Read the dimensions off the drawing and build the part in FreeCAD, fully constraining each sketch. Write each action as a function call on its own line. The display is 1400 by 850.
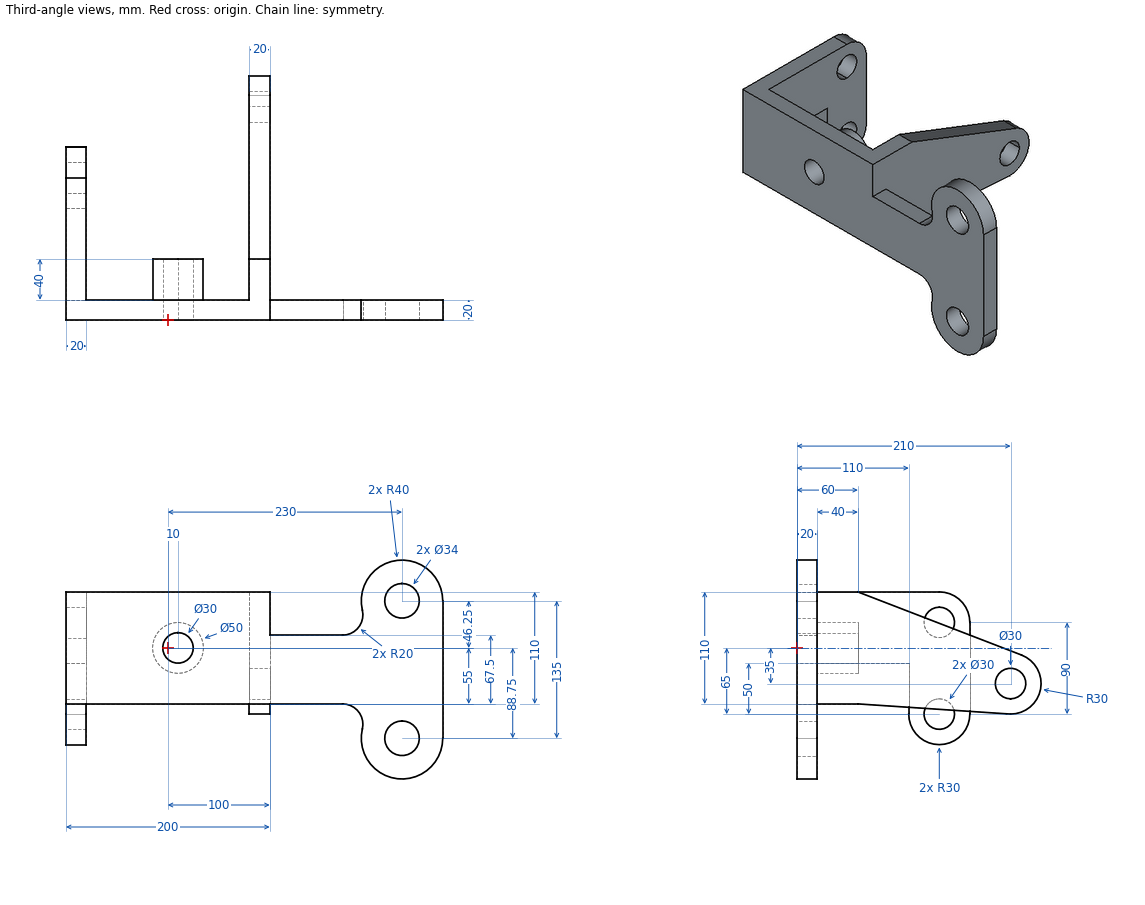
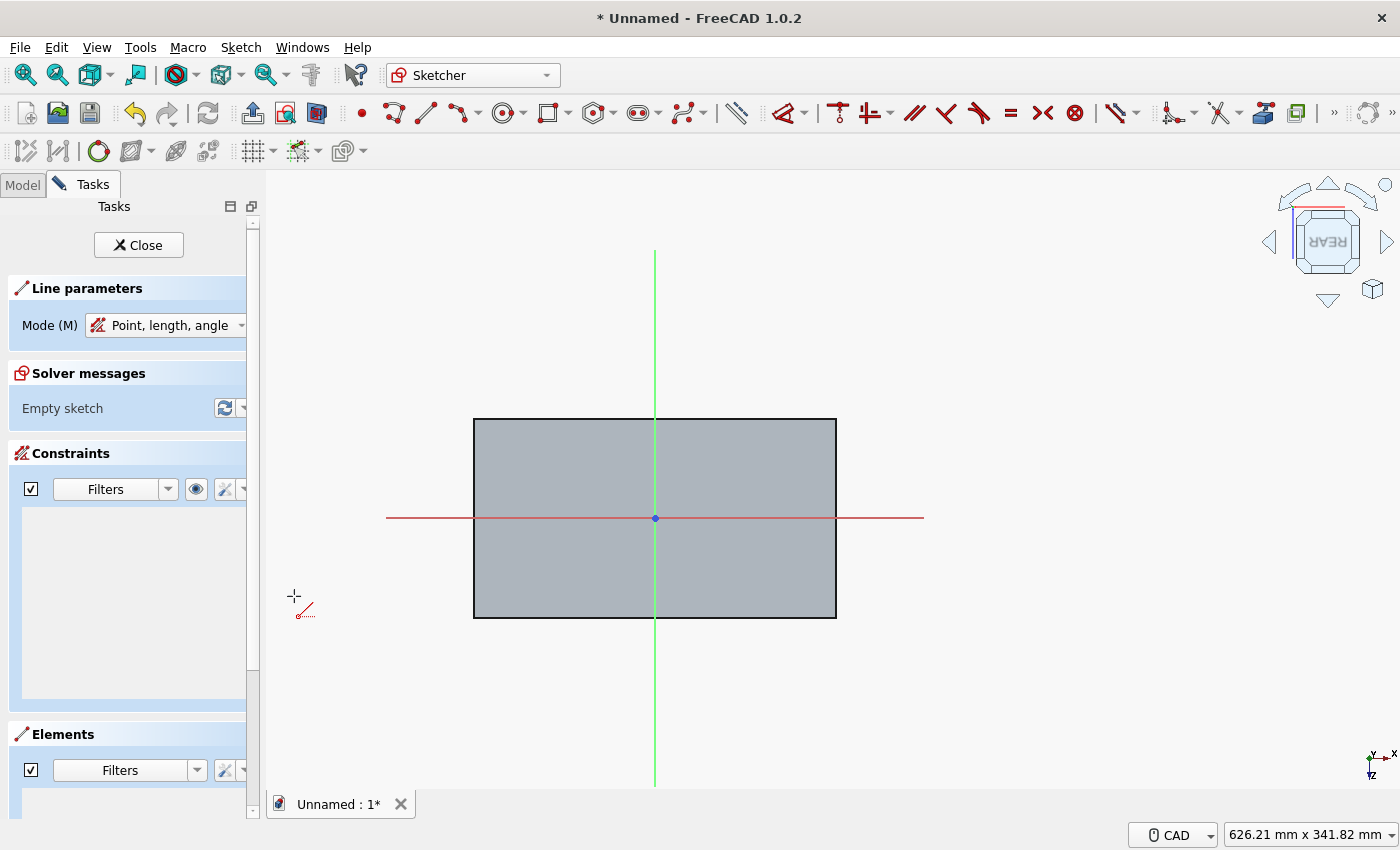
click(1144, 602)
click(1144, 357)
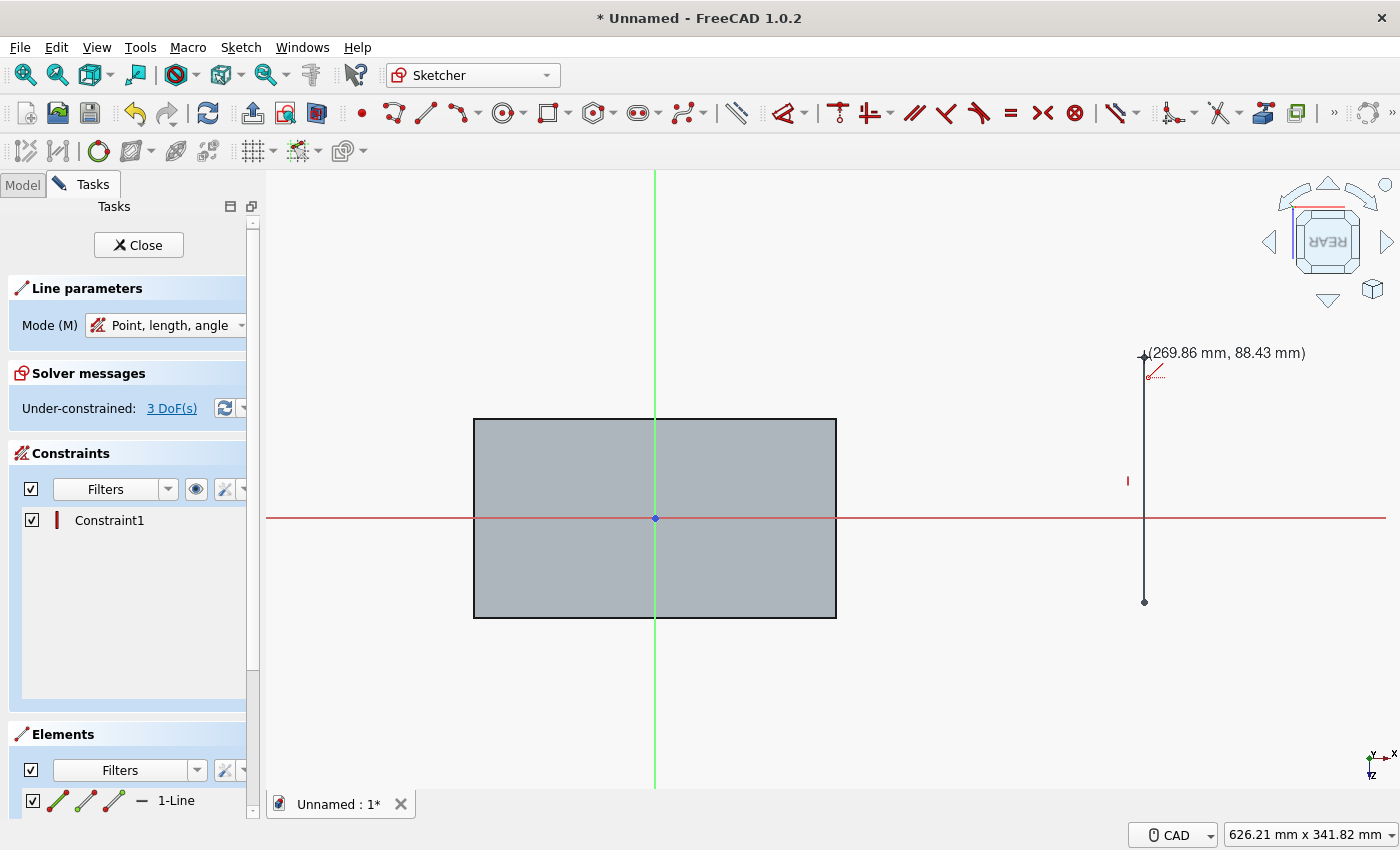
key(g)
key(m)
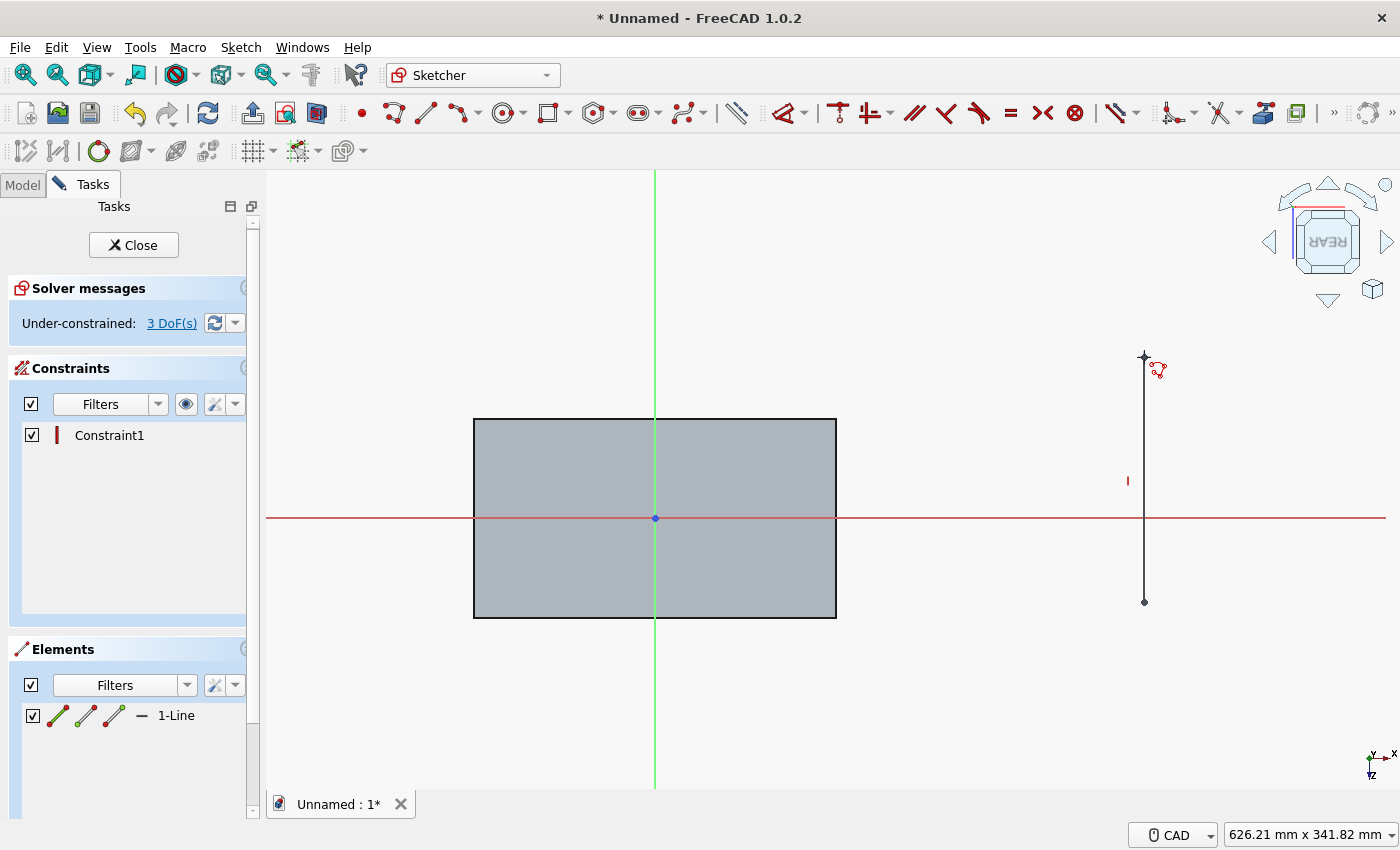
click(966, 419)
click(836, 419)
click(836, 541)
click(966, 541)
right_click(966, 541)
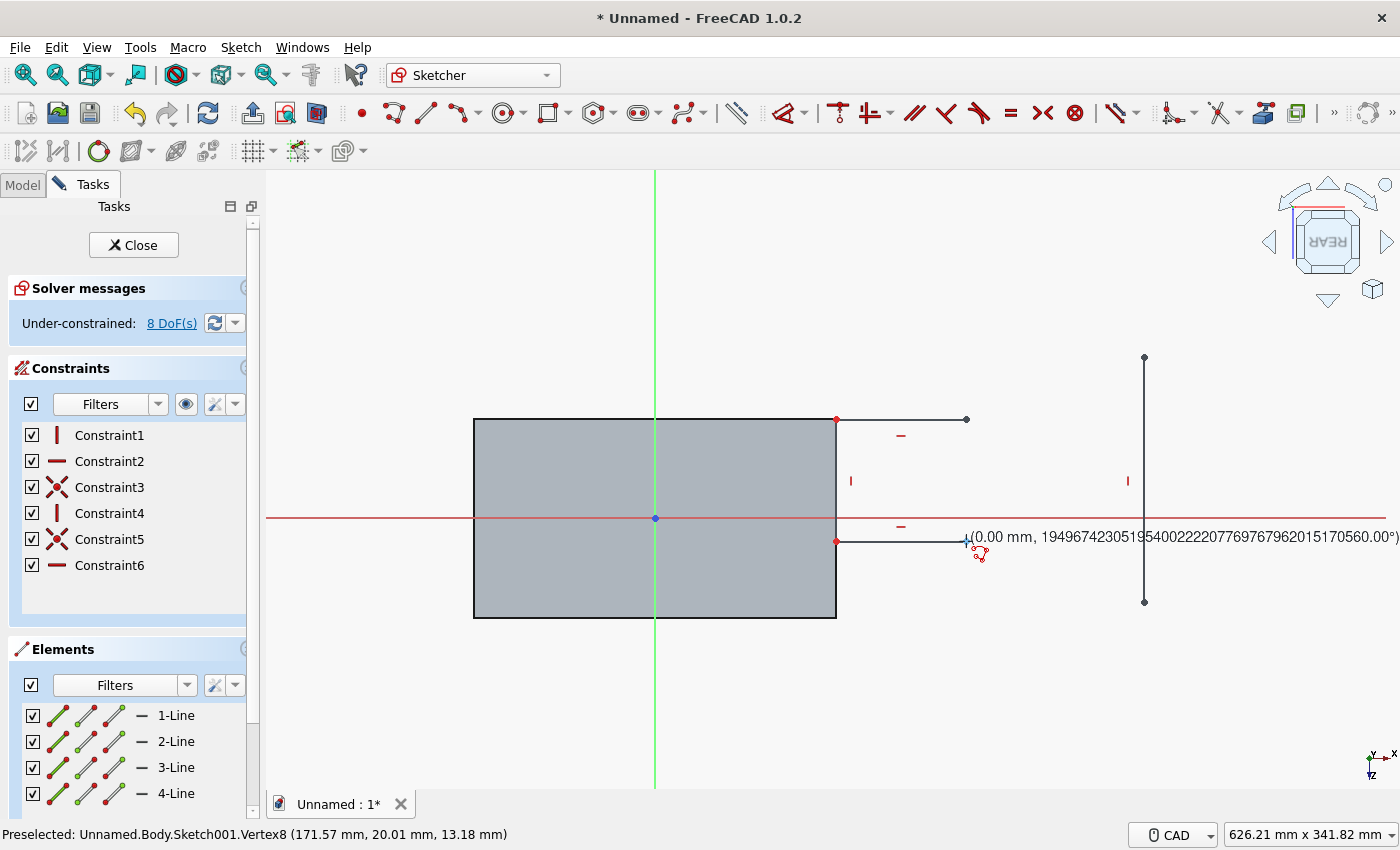
key(g)
key(3)
key(a)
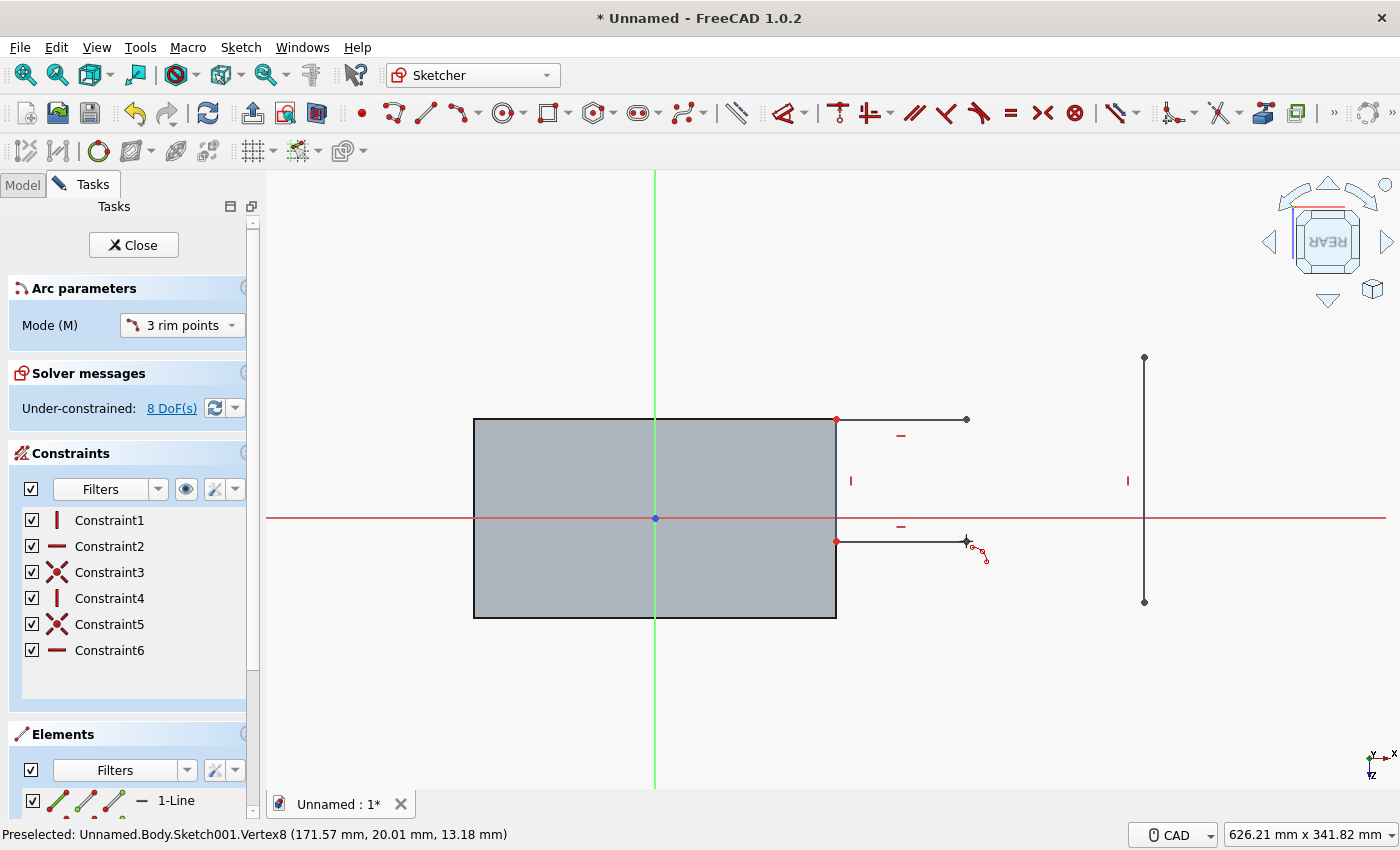
click(1144, 358)
click(1001, 374)
click(1063, 285)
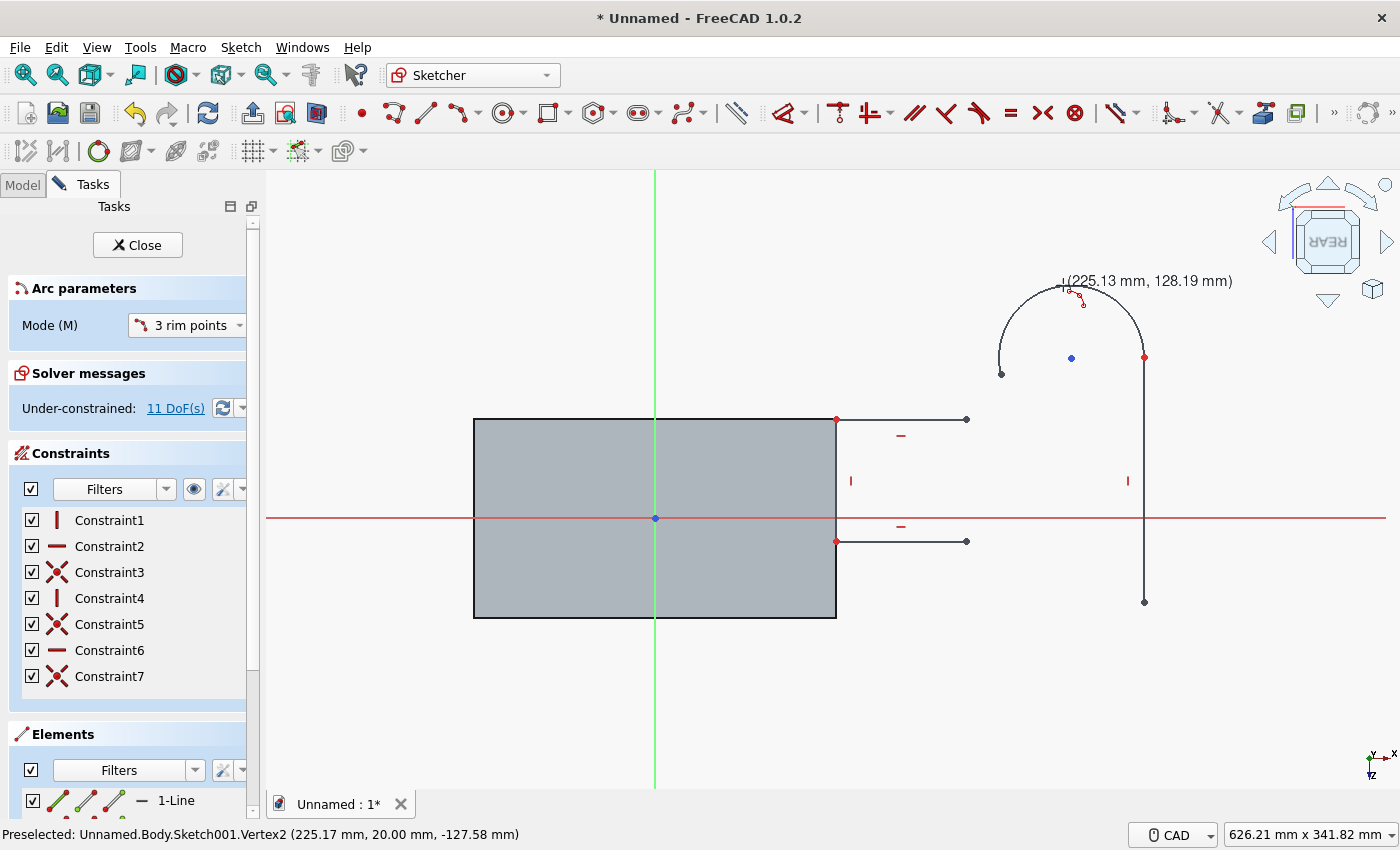
click(1001, 375)
click(966, 420)
click(994, 405)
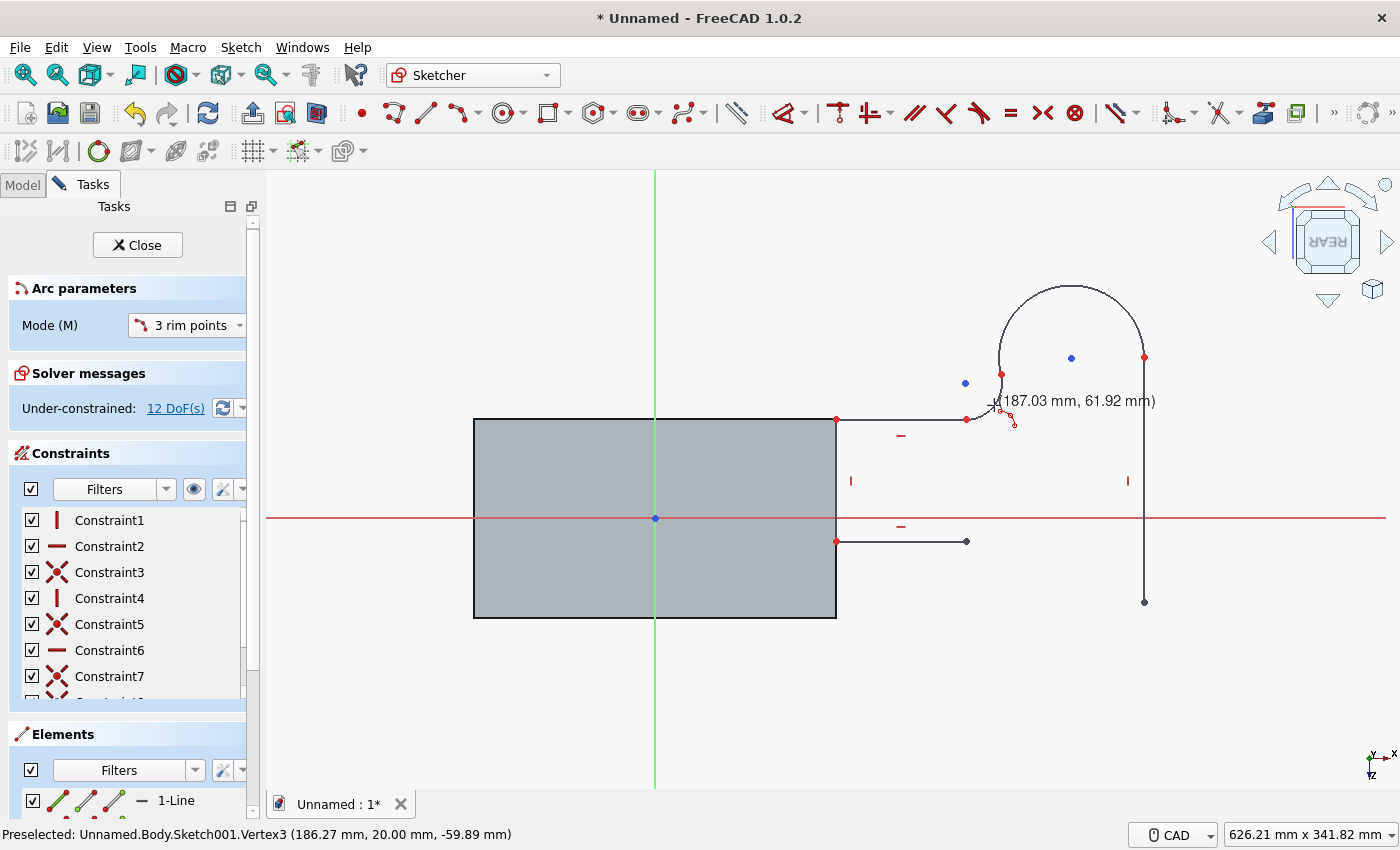
click(966, 542)
click(1001, 585)
click(994, 555)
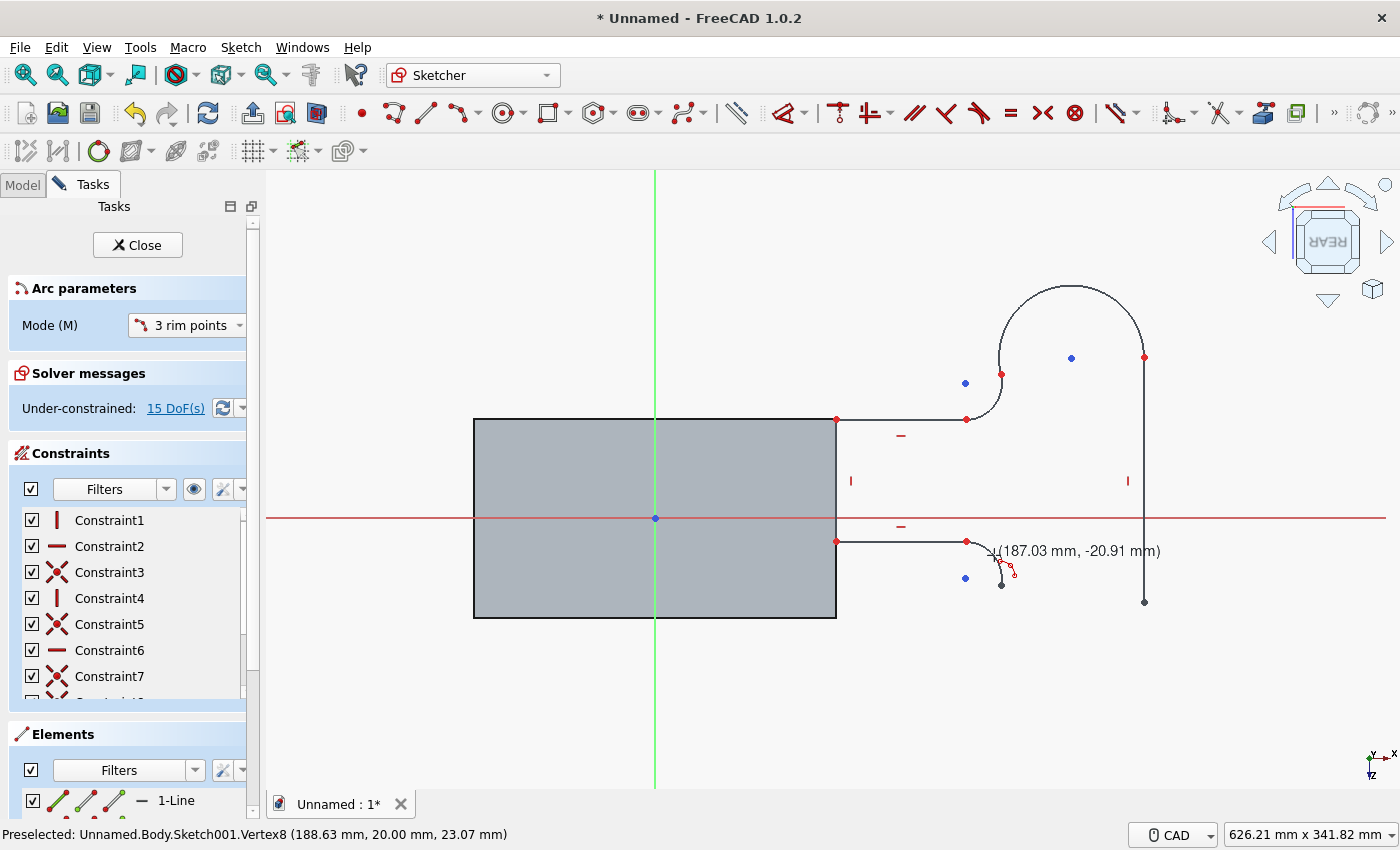
click(1001, 586)
click(1144, 603)
click(1063, 674)